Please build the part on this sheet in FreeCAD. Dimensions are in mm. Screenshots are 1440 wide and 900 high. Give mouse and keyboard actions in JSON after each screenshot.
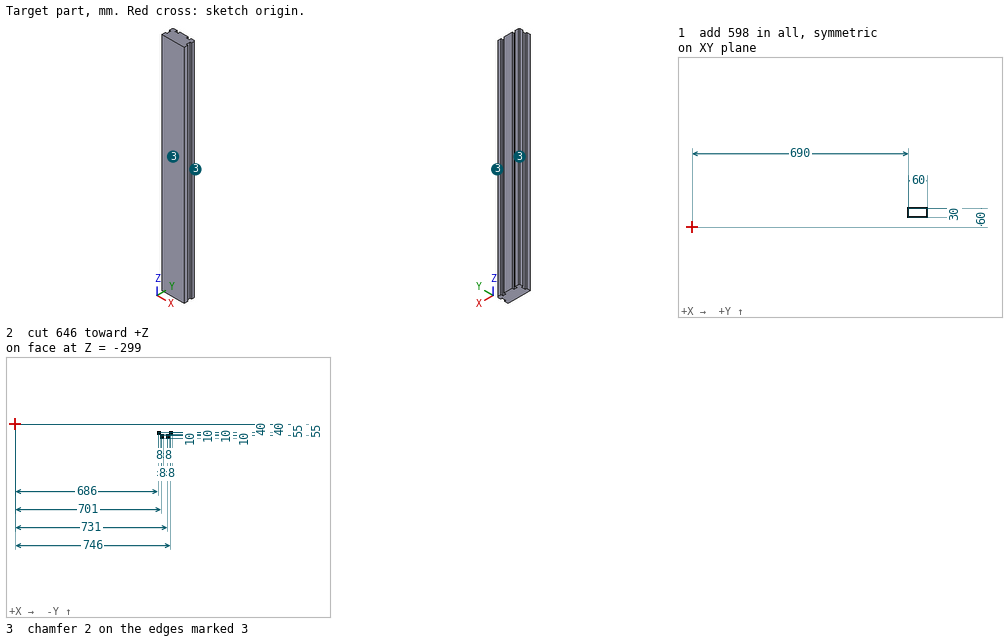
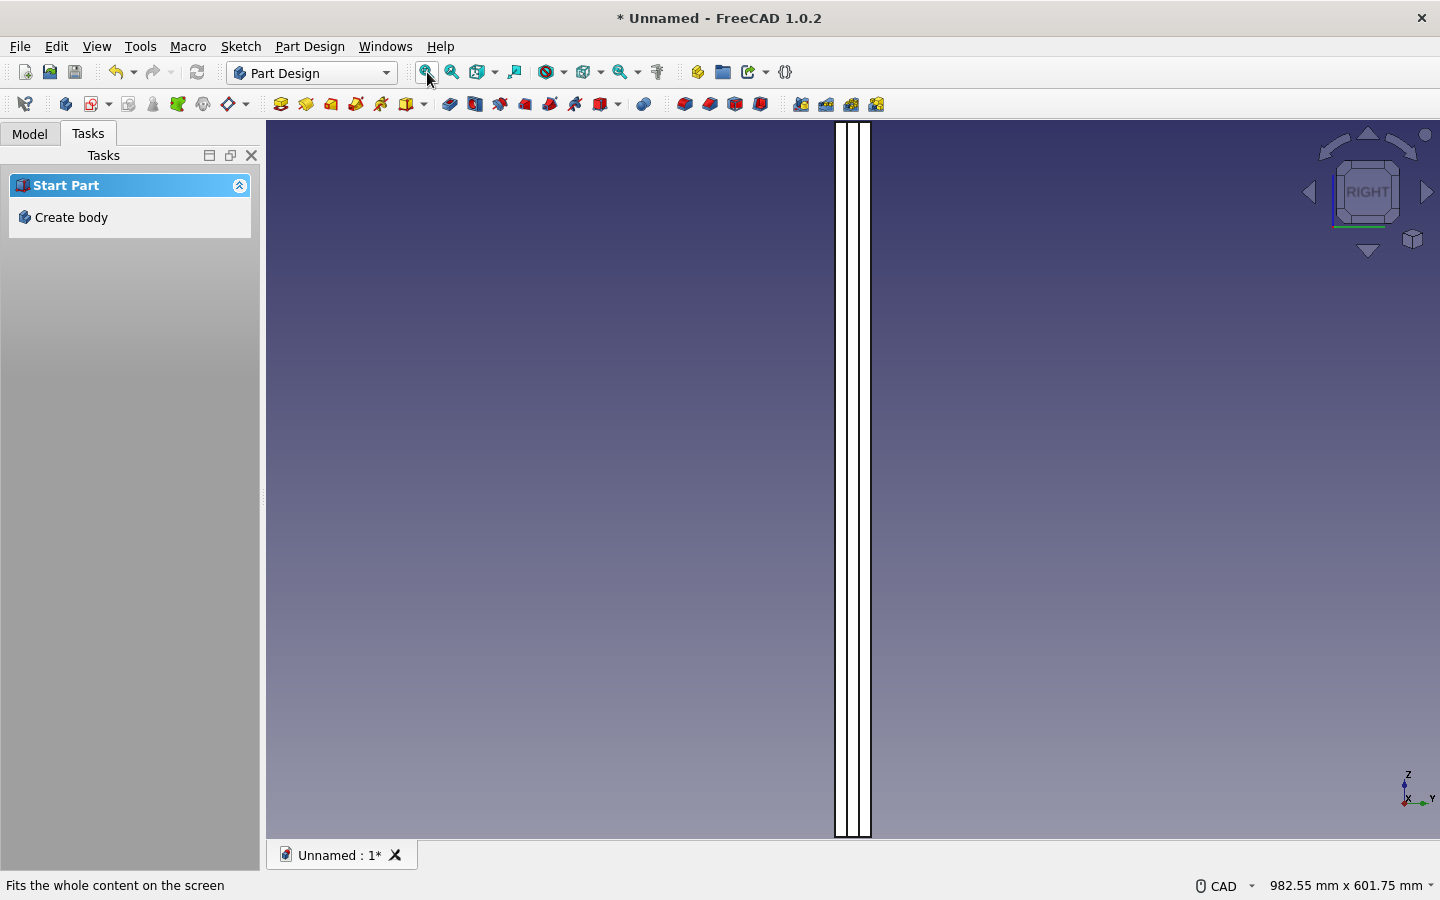
{"action": "left_click", "coordinate": [871, 479]}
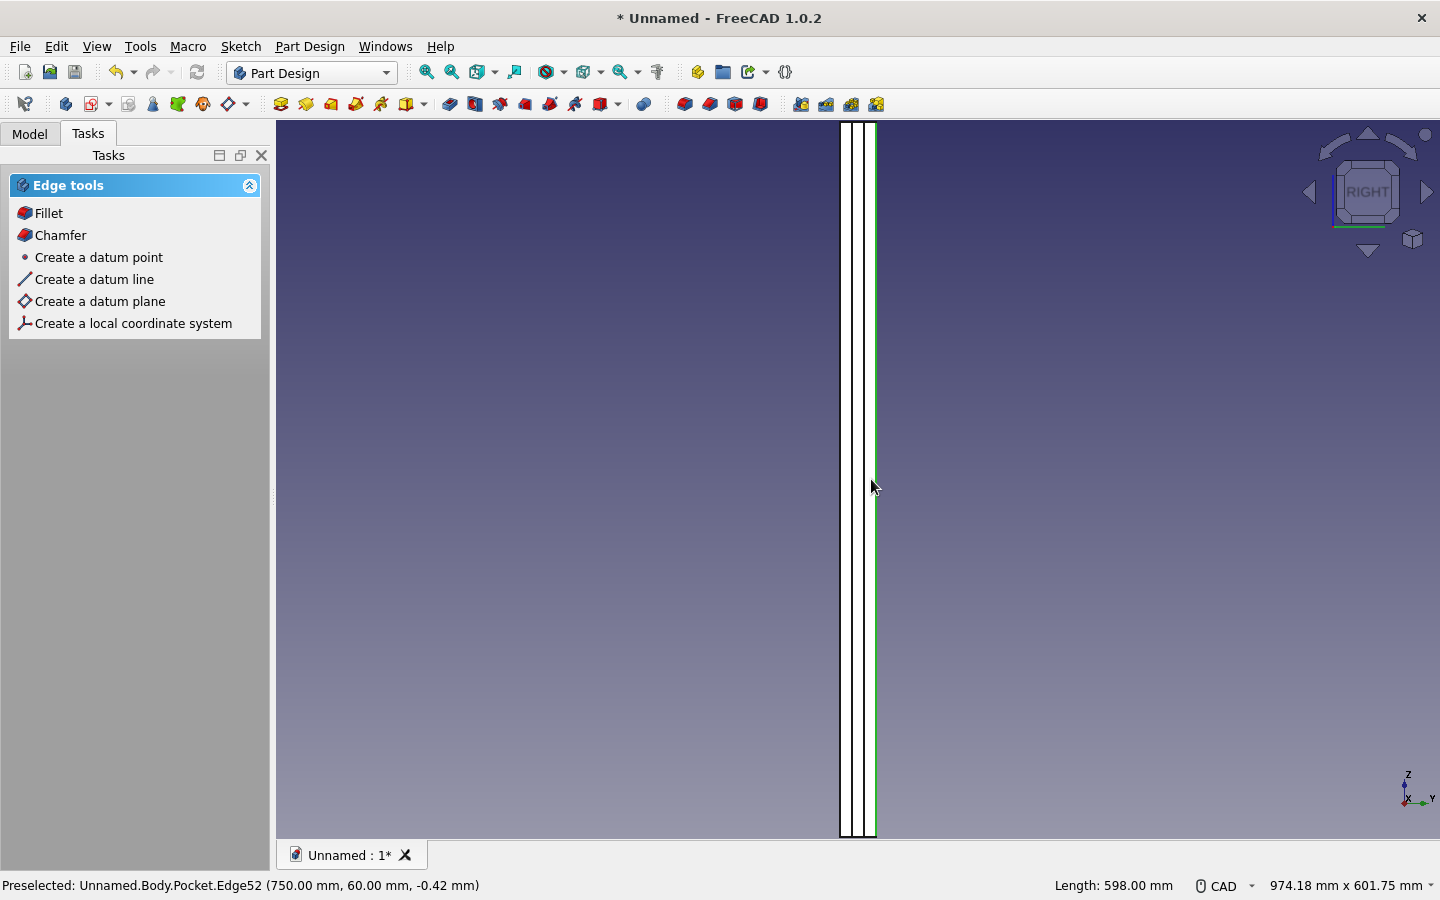
{"action": "key", "text": "5"}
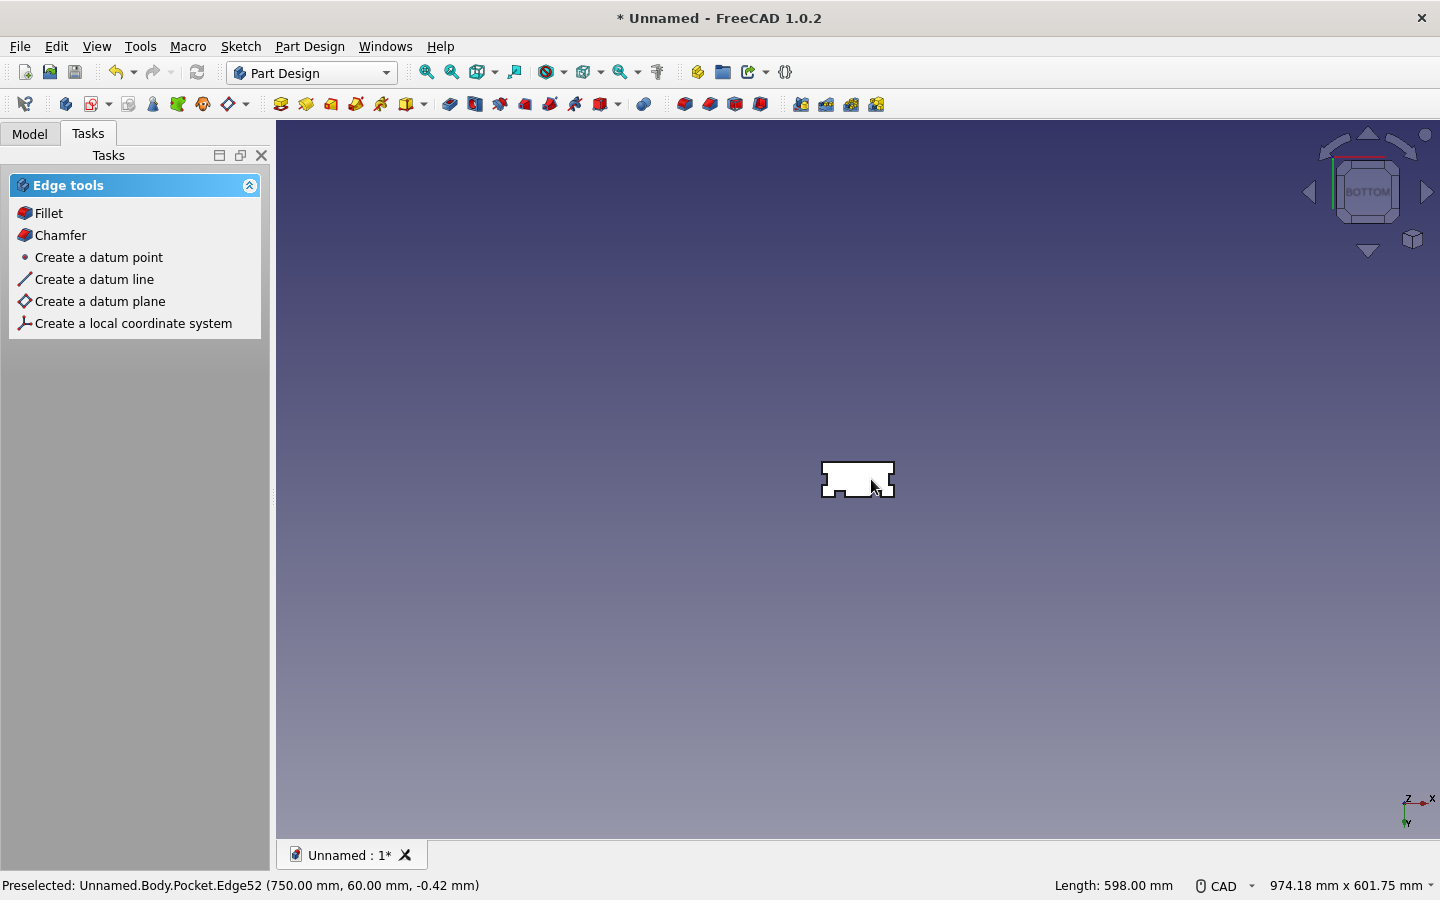
{"action": "left_click", "coordinate": [427, 72]}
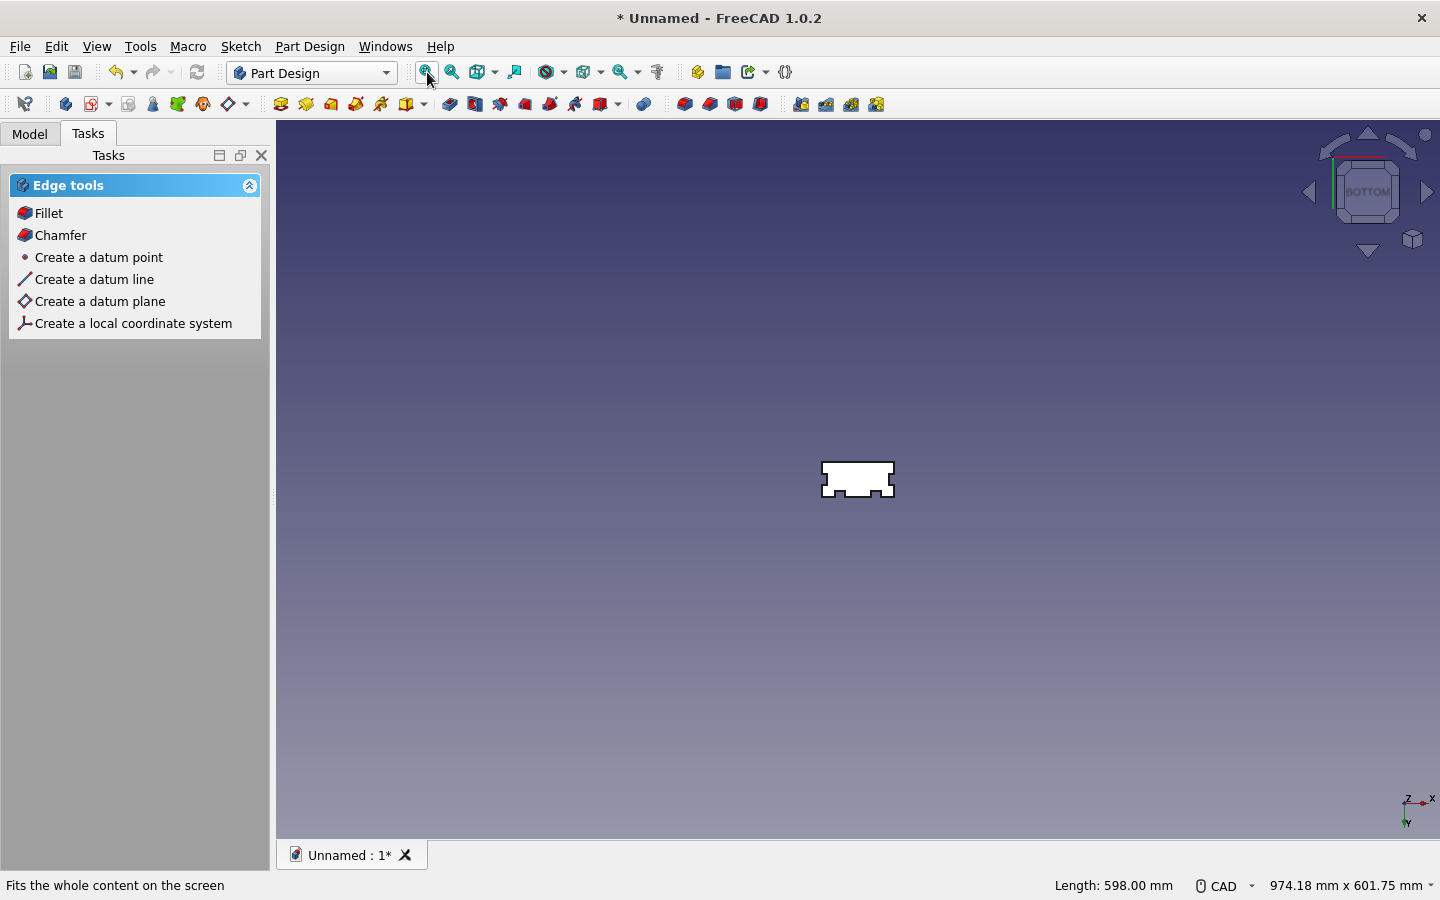
{"action": "key", "text": "4"}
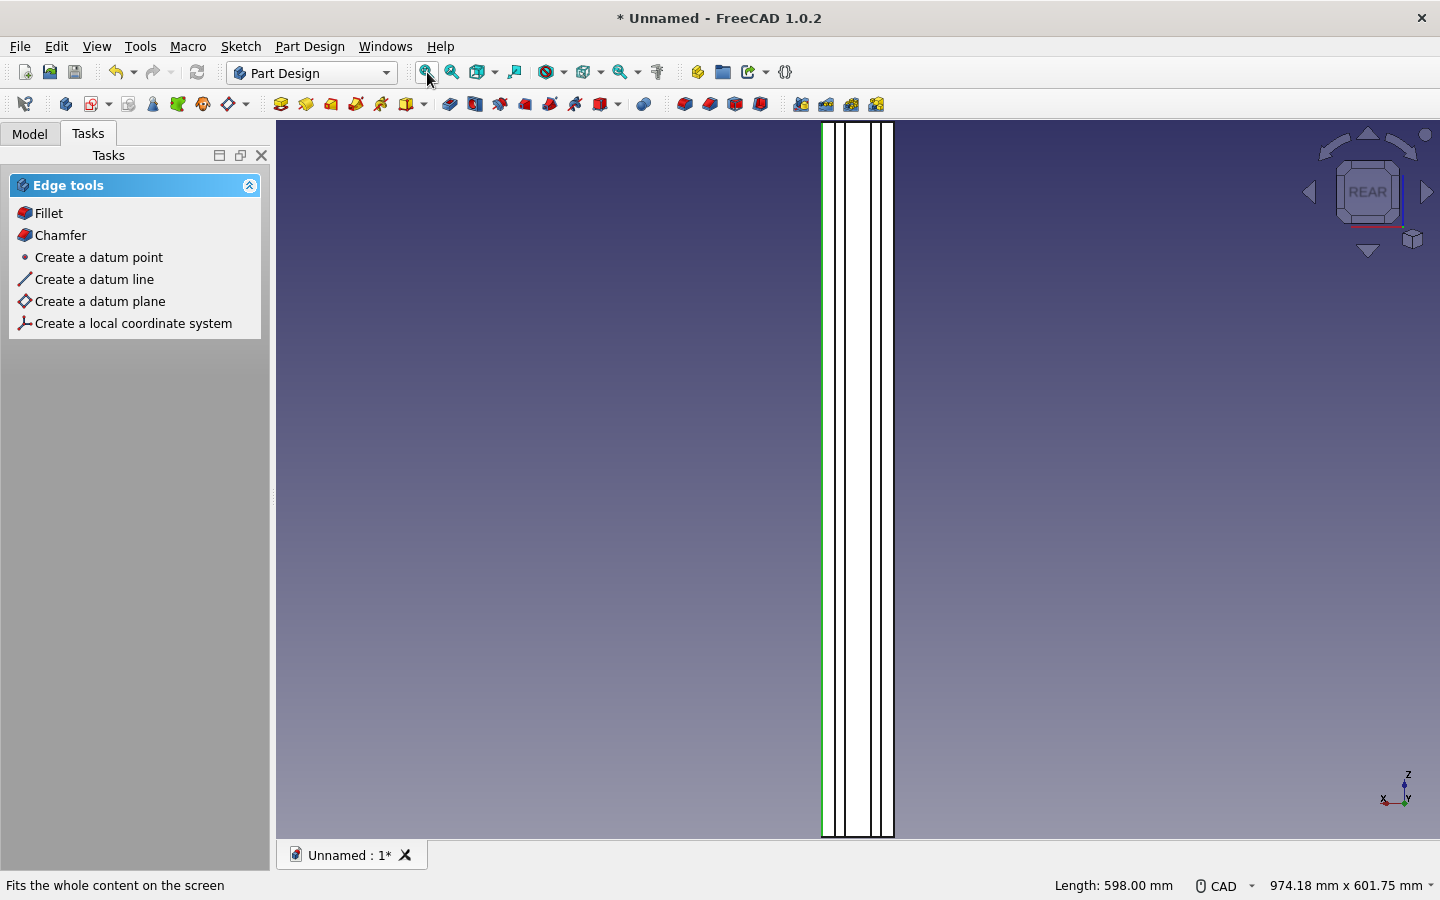
{"action": "left_click", "coordinate": [894, 479], "text": "ctrl"}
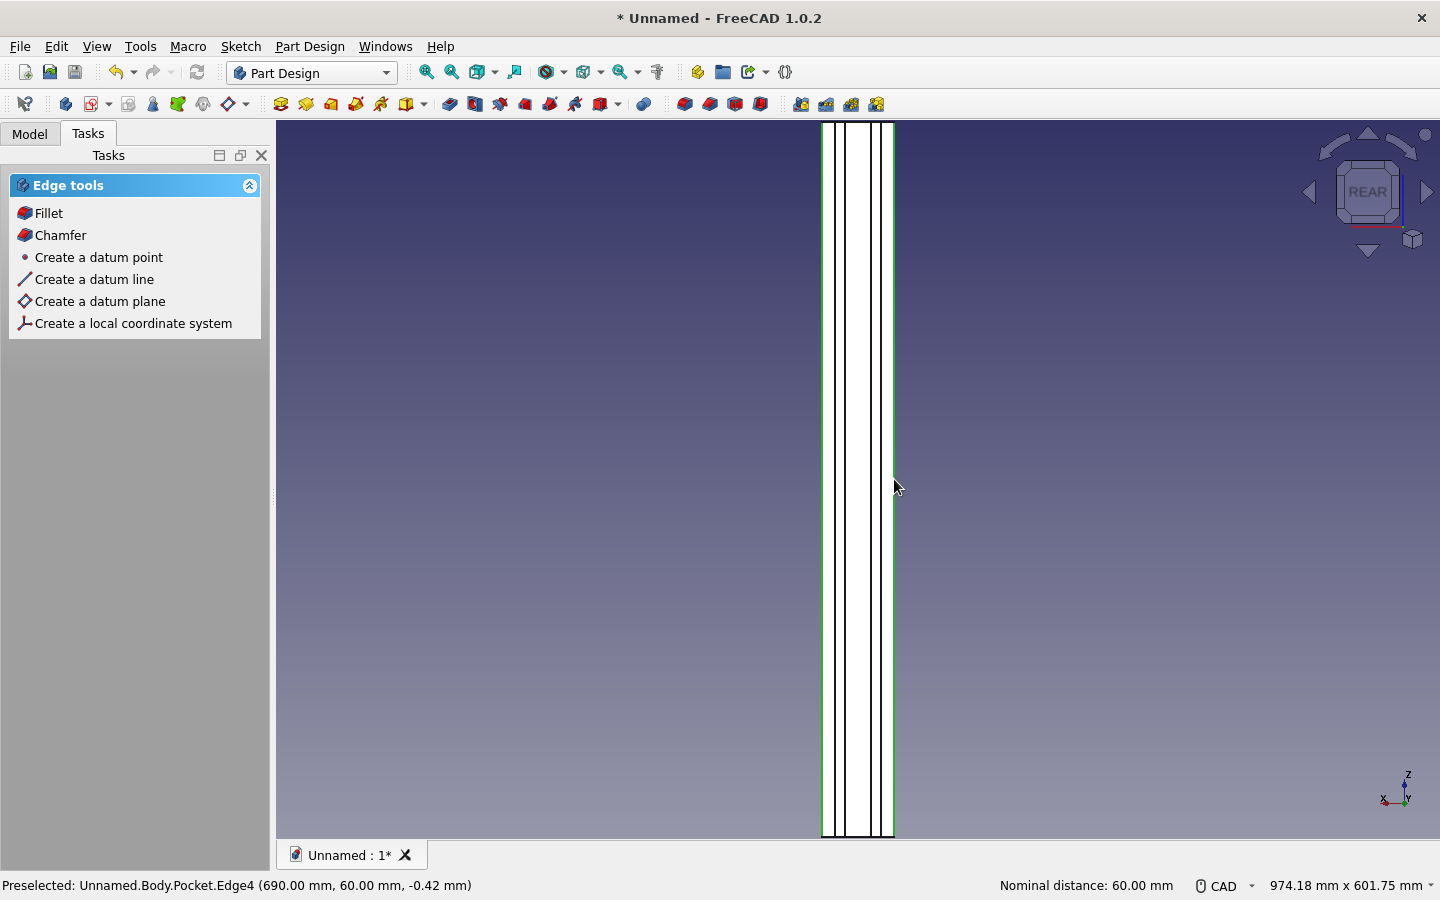
{"action": "left_click", "coordinate": [710, 104]}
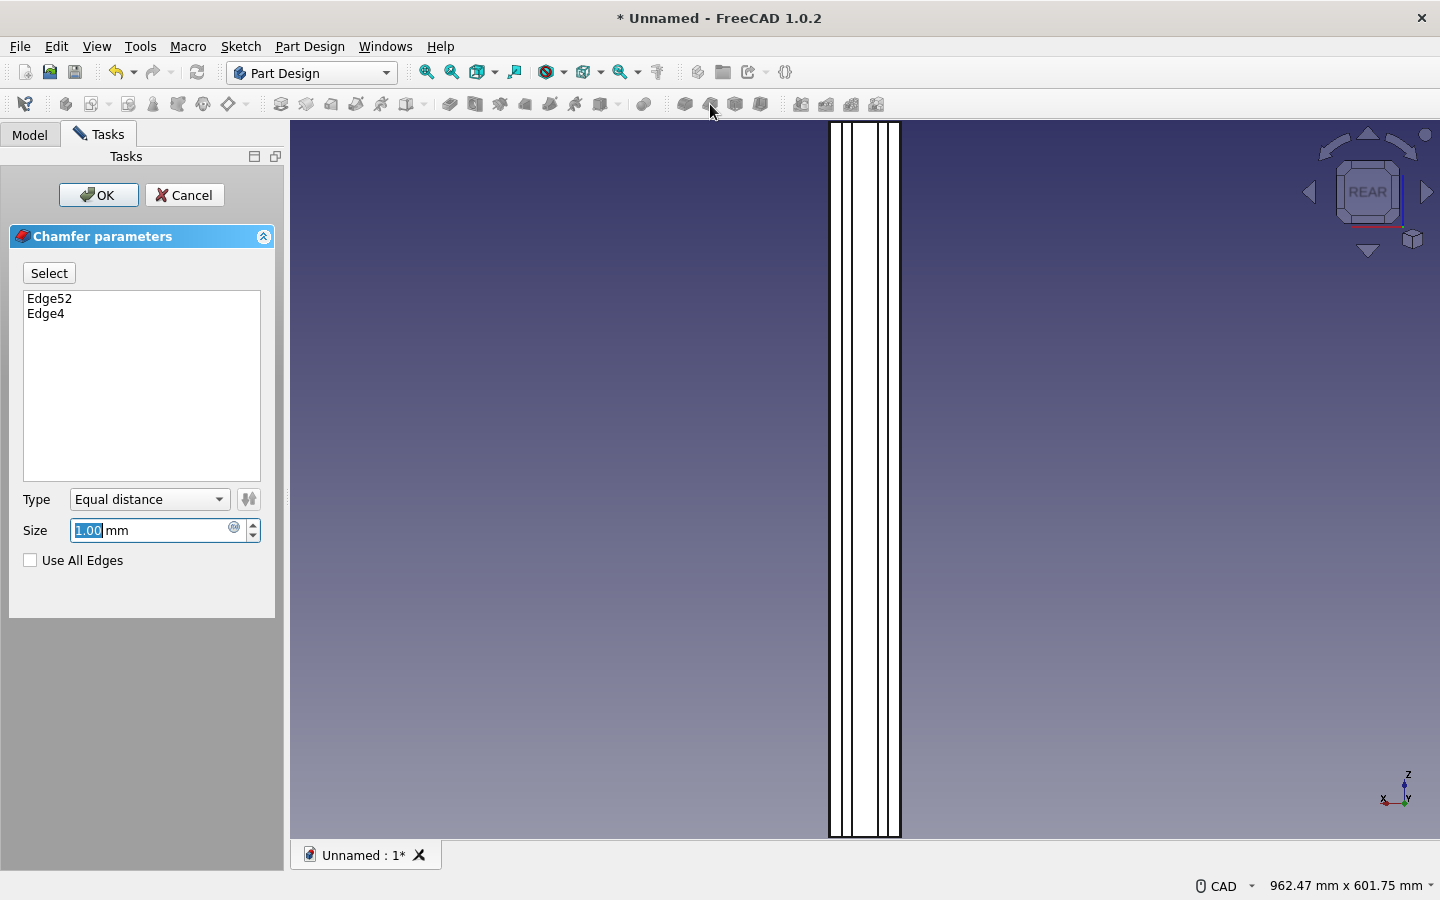
{"action": "type", "text": "2"}
{"action": "key", "text": "Tab"}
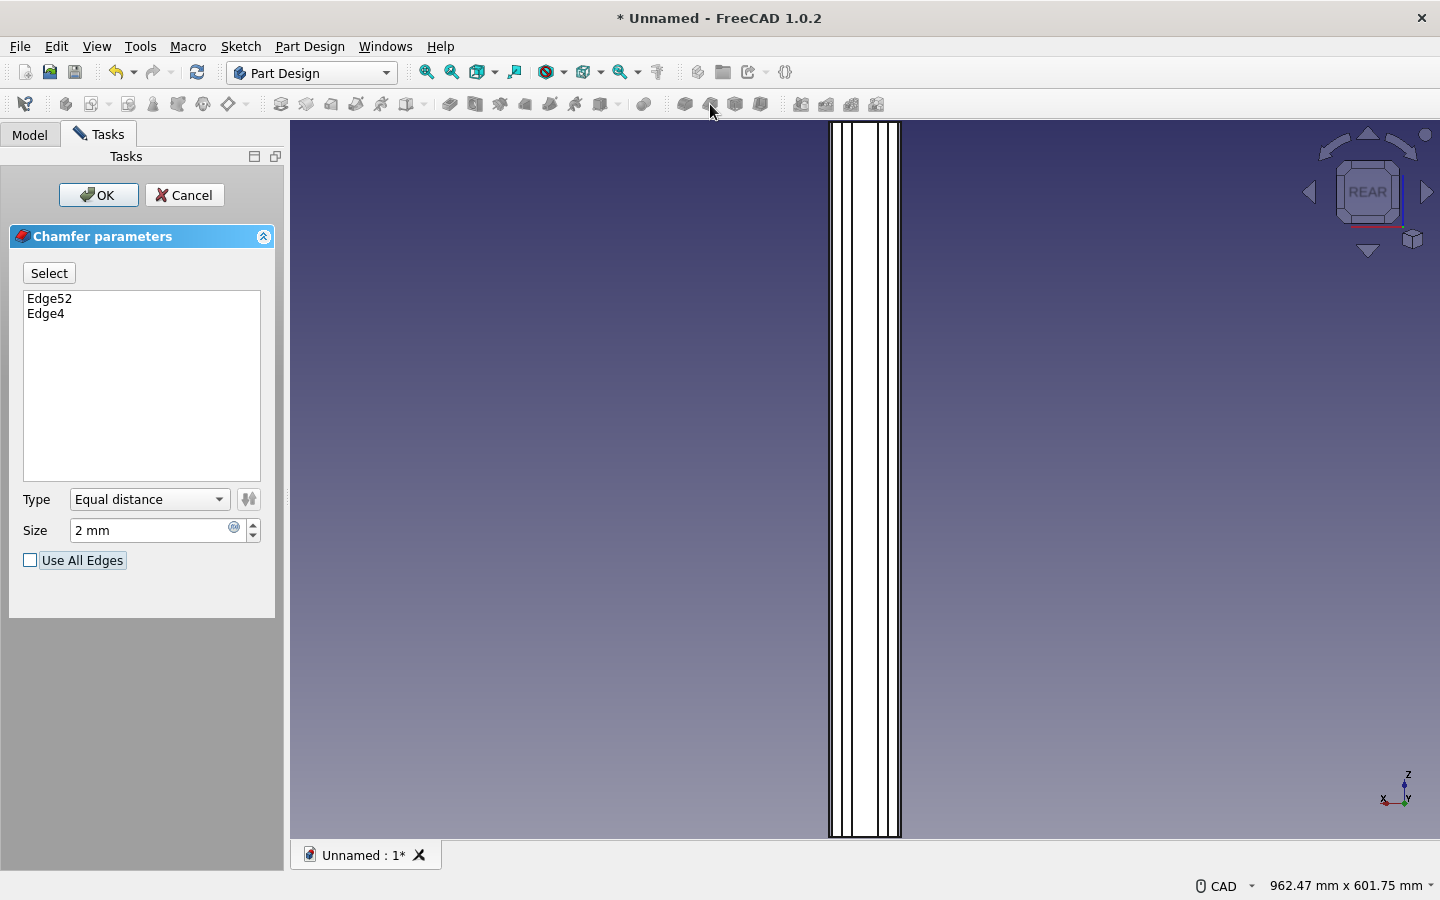
{"action": "left_click", "coordinate": [99, 195]}